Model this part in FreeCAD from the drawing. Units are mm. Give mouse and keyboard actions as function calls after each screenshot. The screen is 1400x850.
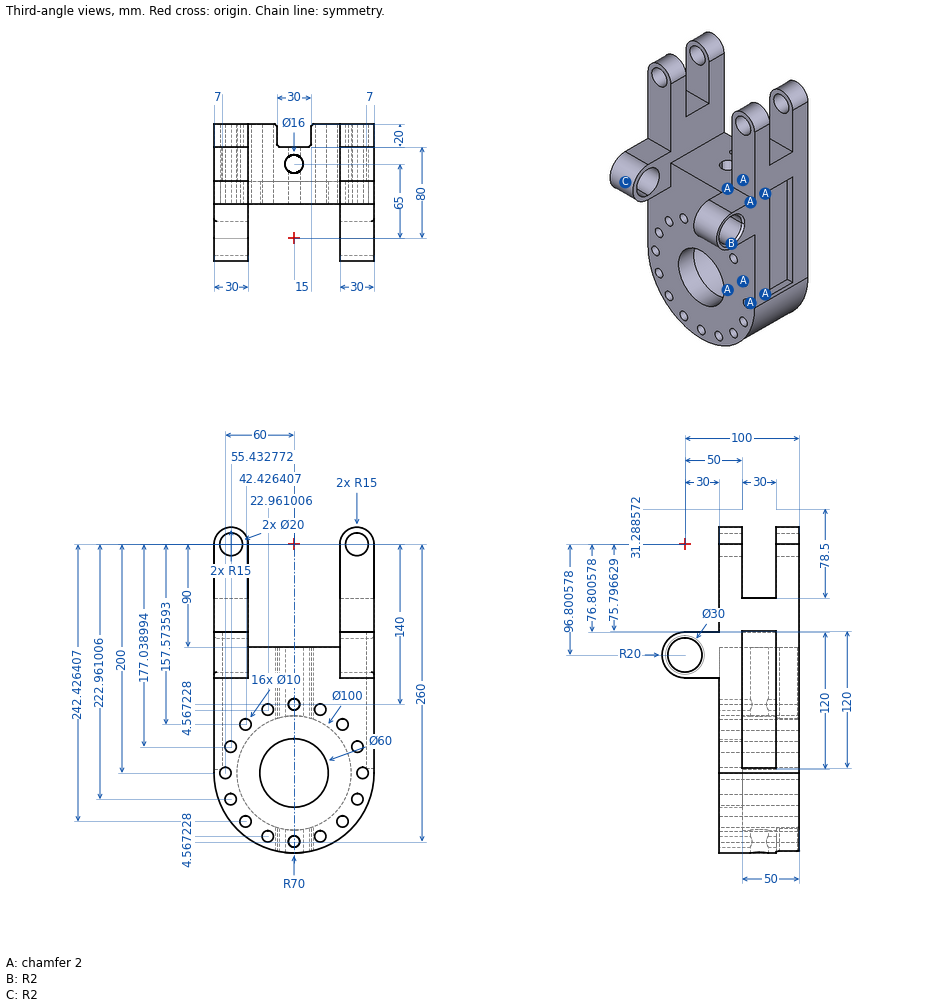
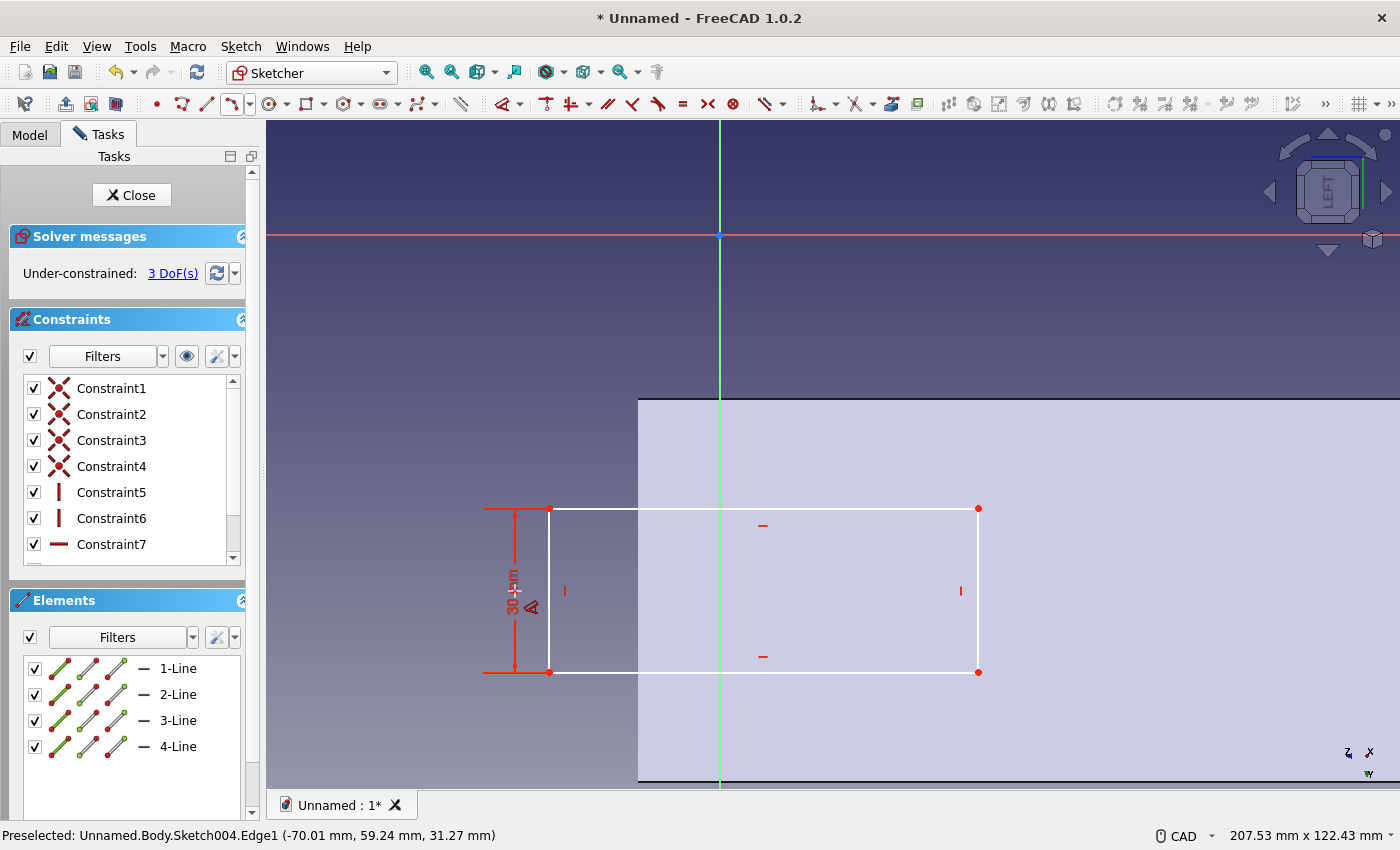
click(549, 509)
click(515, 372)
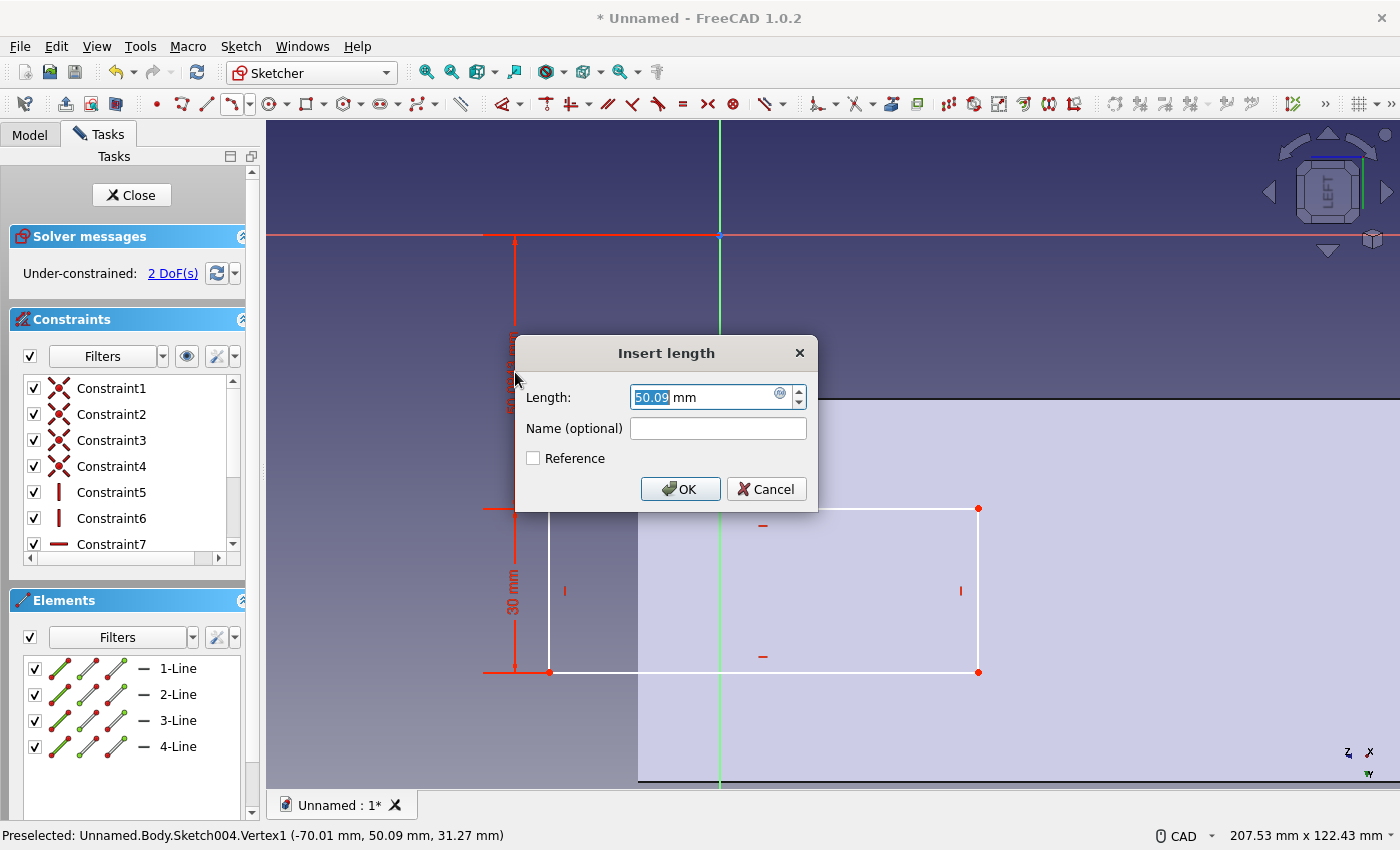
text(50)
key(Return)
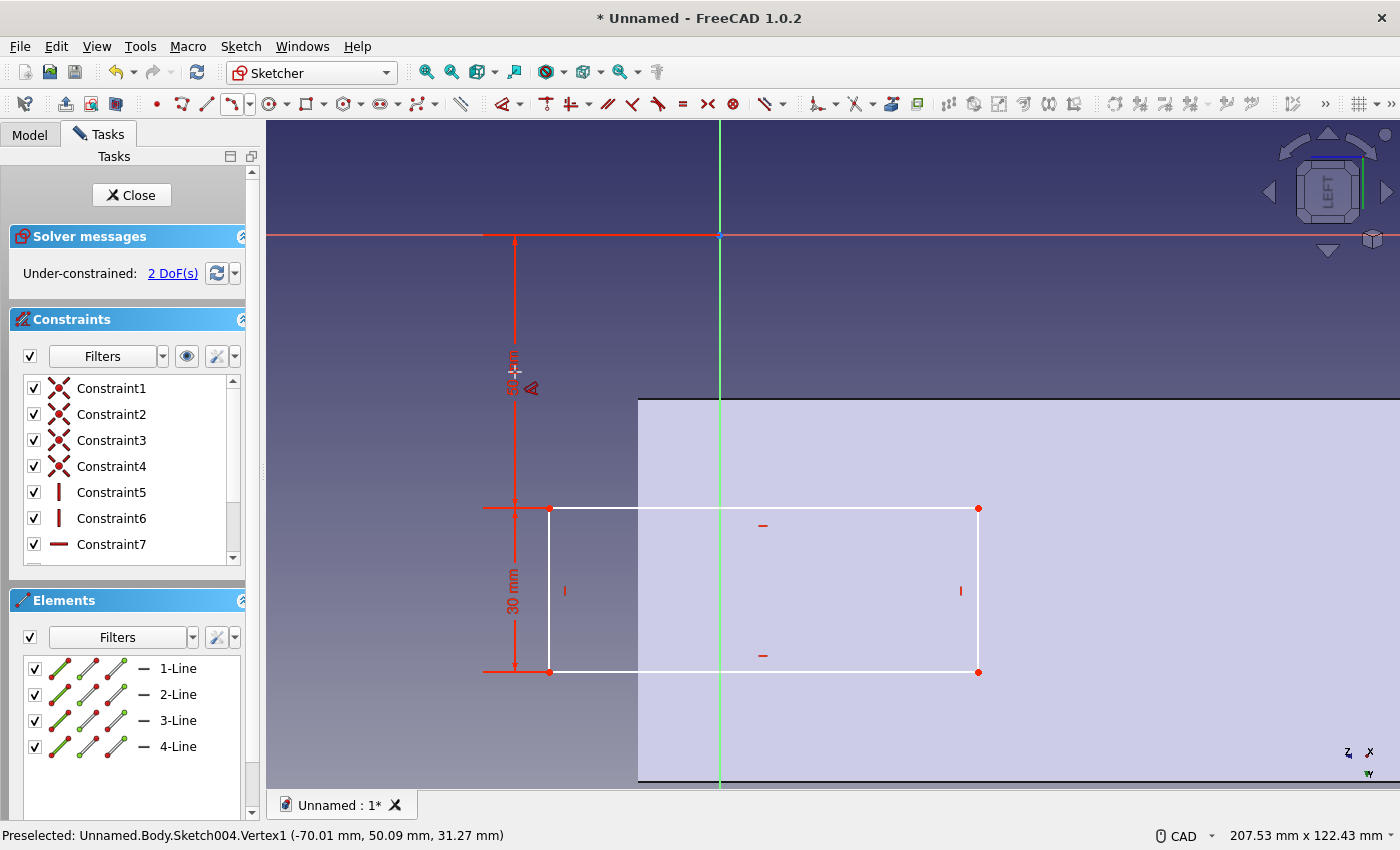
click(678, 672)
click(764, 706)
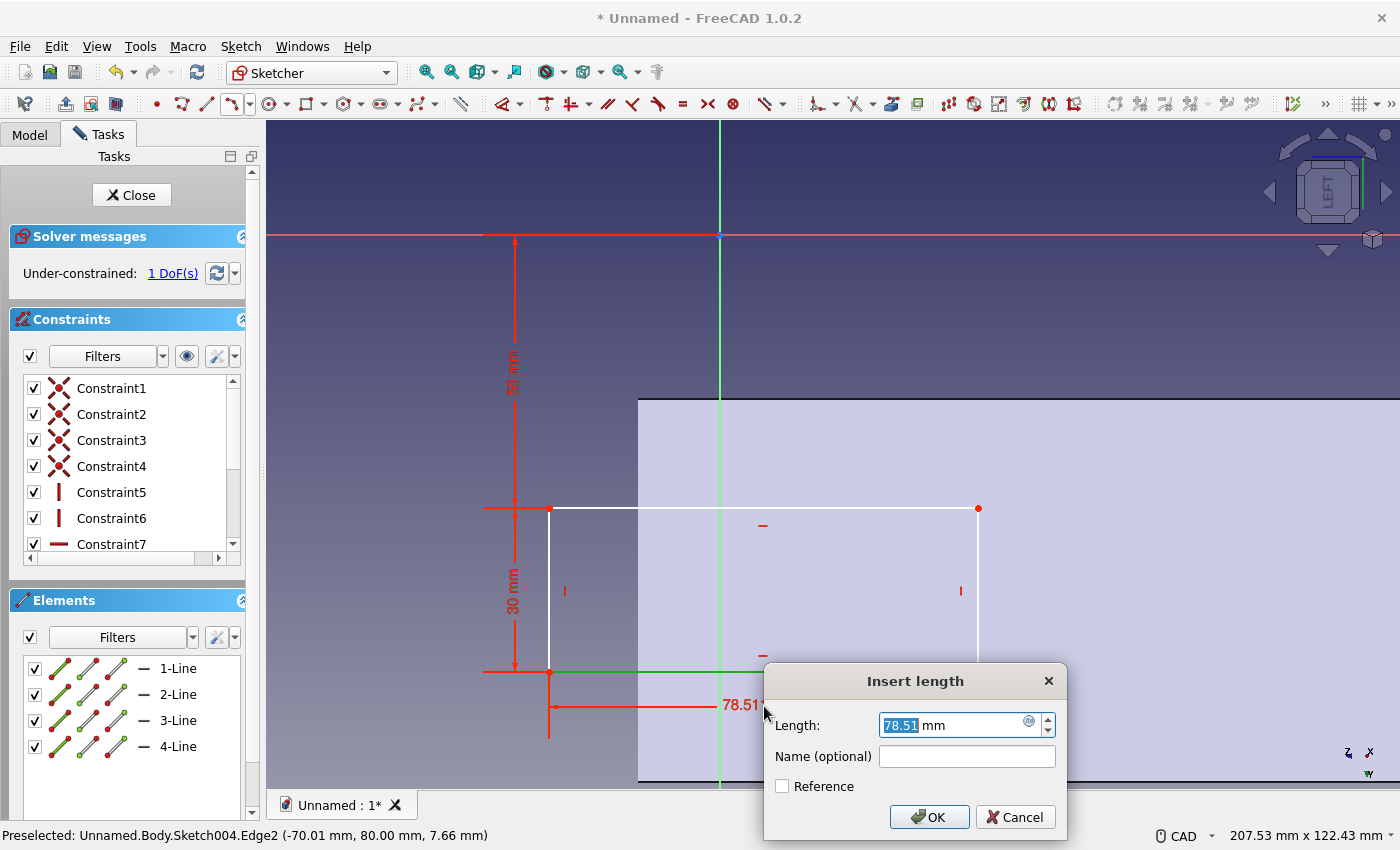
text(78.5)
key(Return)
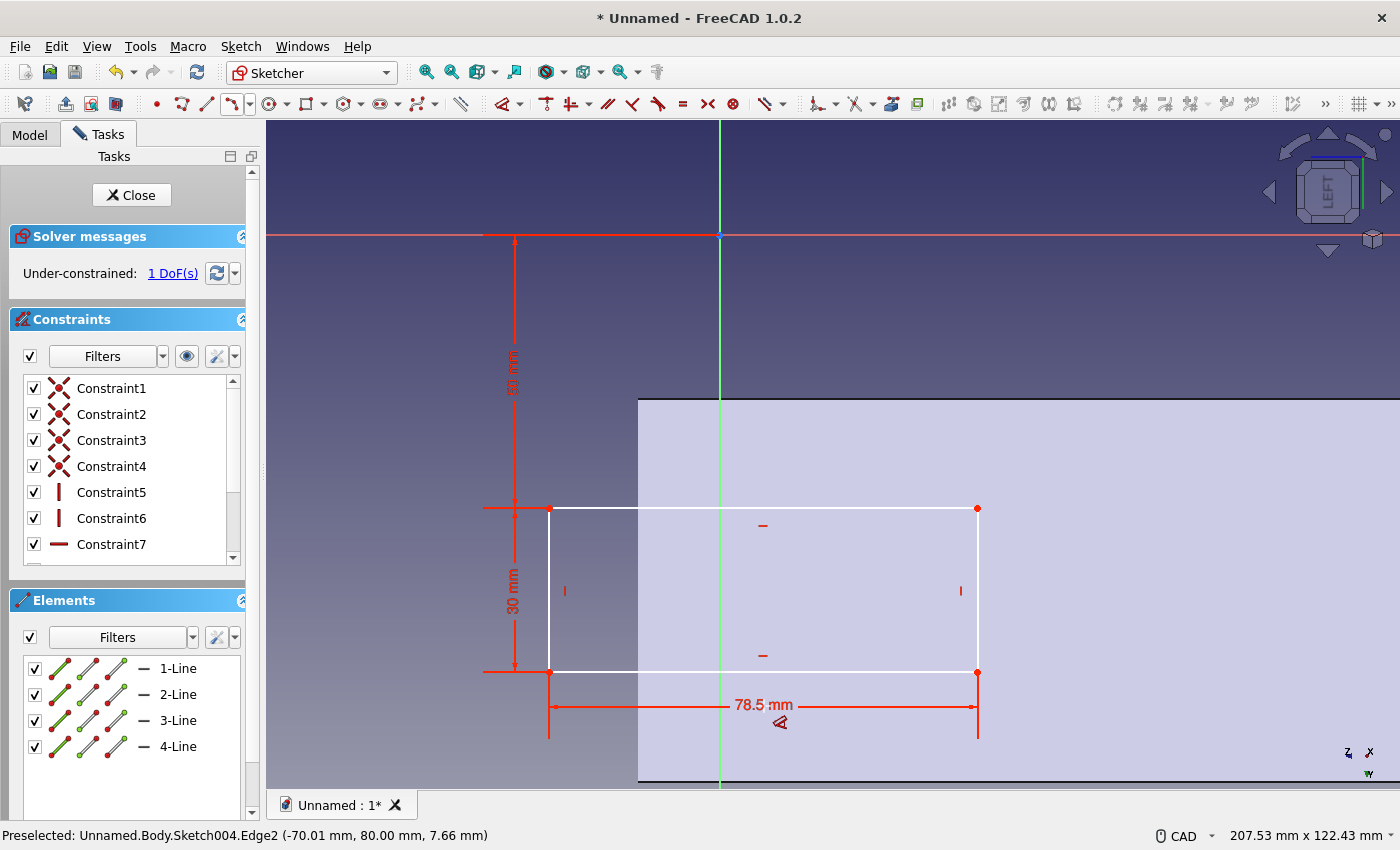
click(549, 508)
click(634, 201)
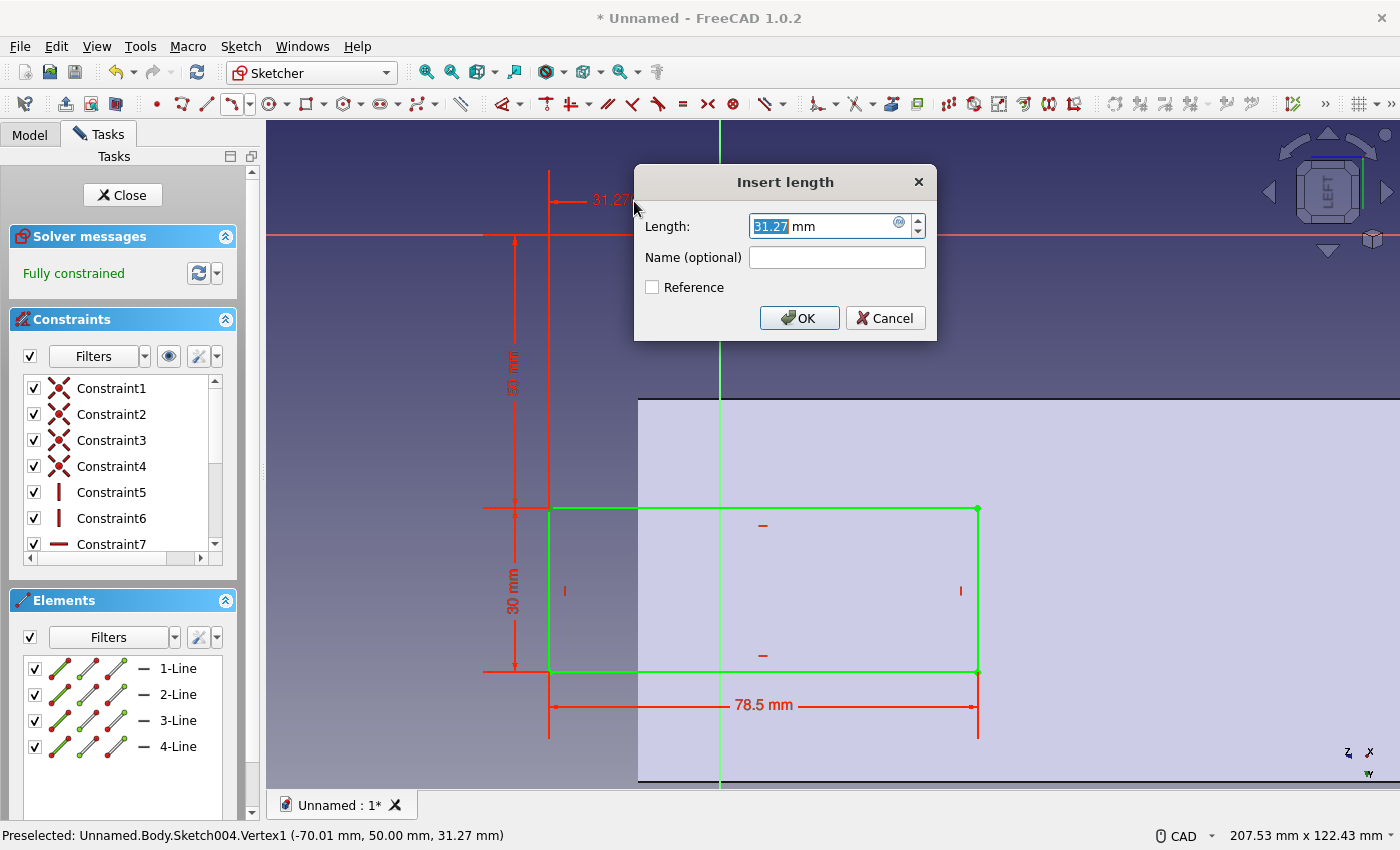
text(31.288572)
key(Return)
key(Escape)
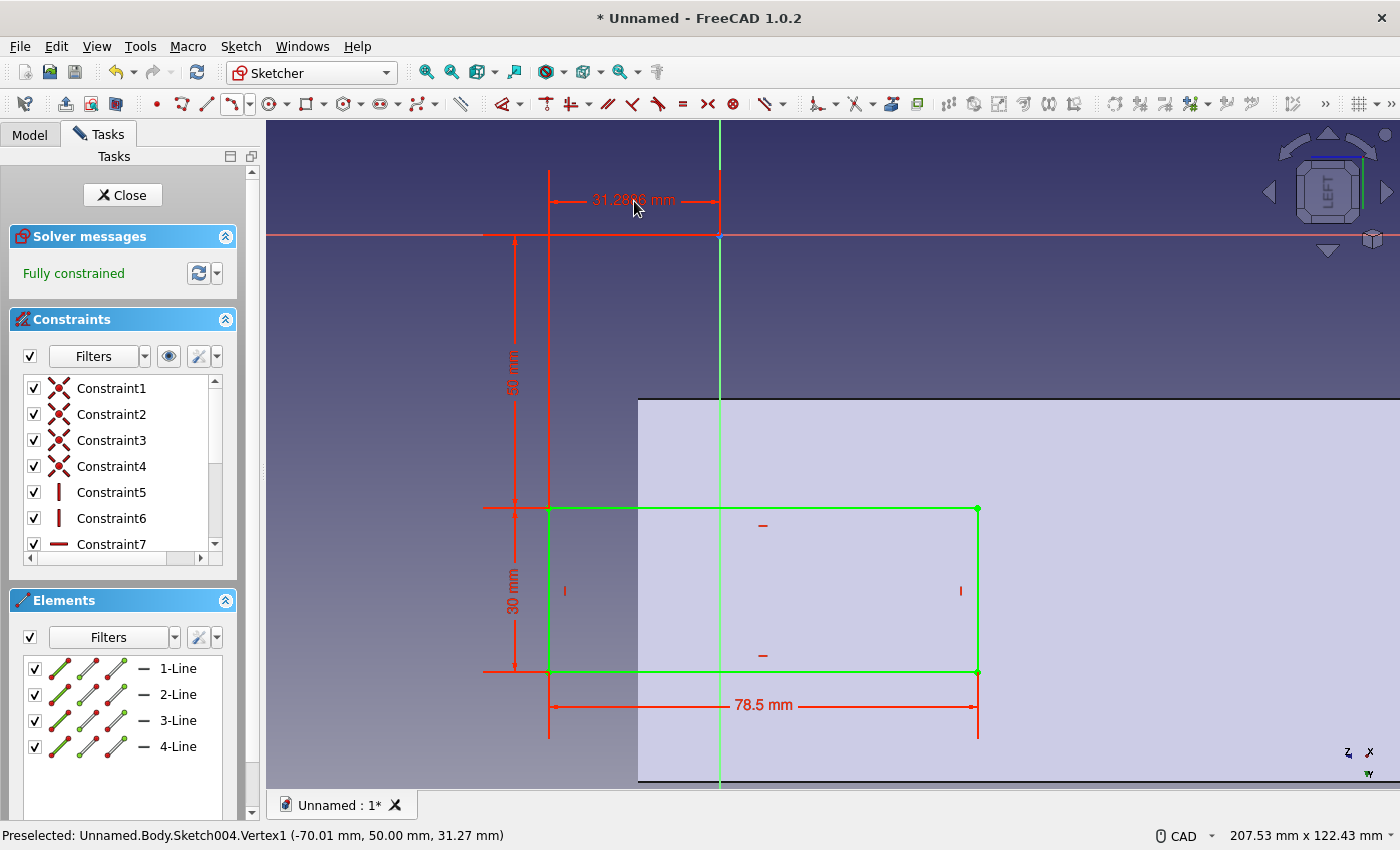
click(123, 195)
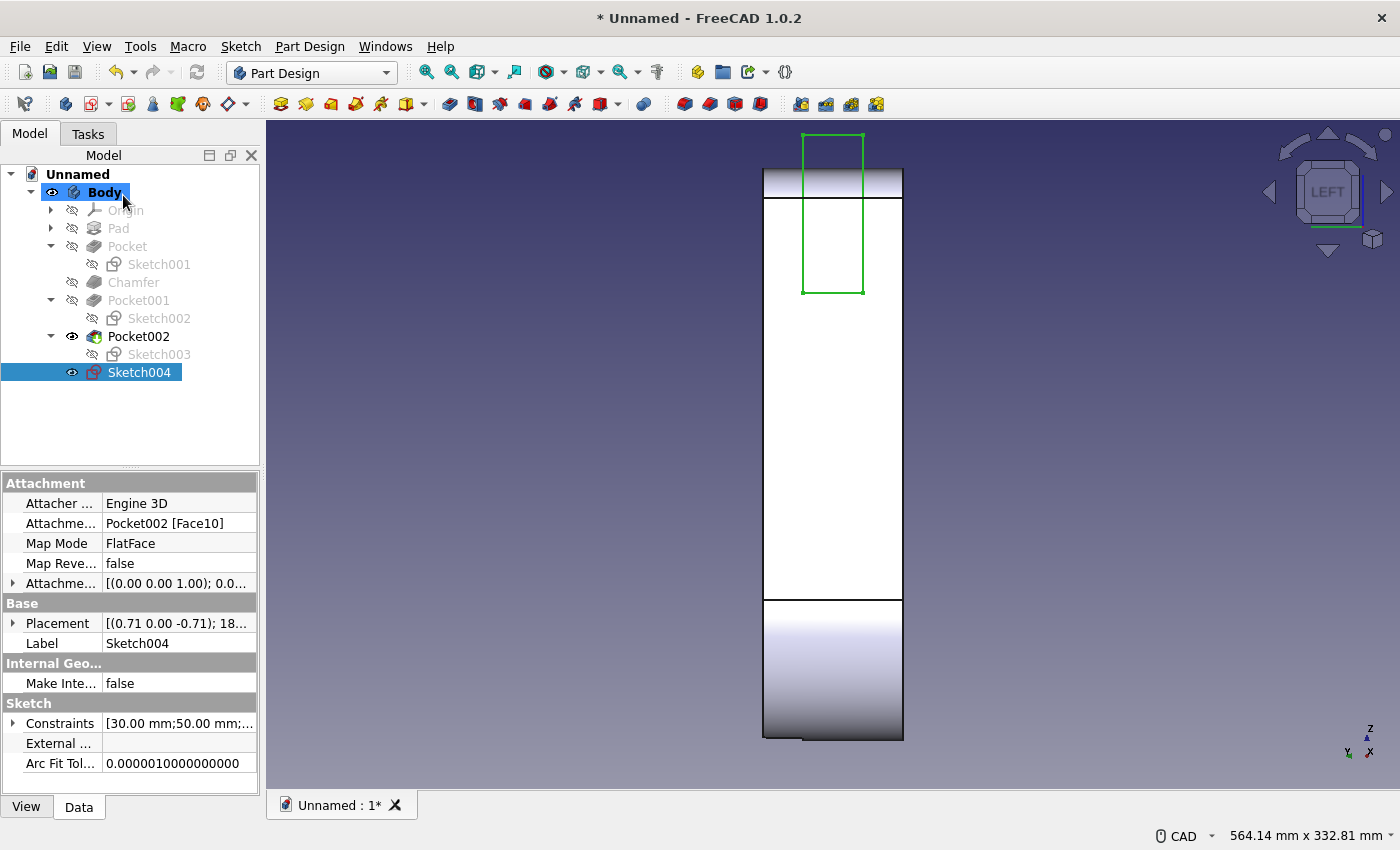
click(450, 104)